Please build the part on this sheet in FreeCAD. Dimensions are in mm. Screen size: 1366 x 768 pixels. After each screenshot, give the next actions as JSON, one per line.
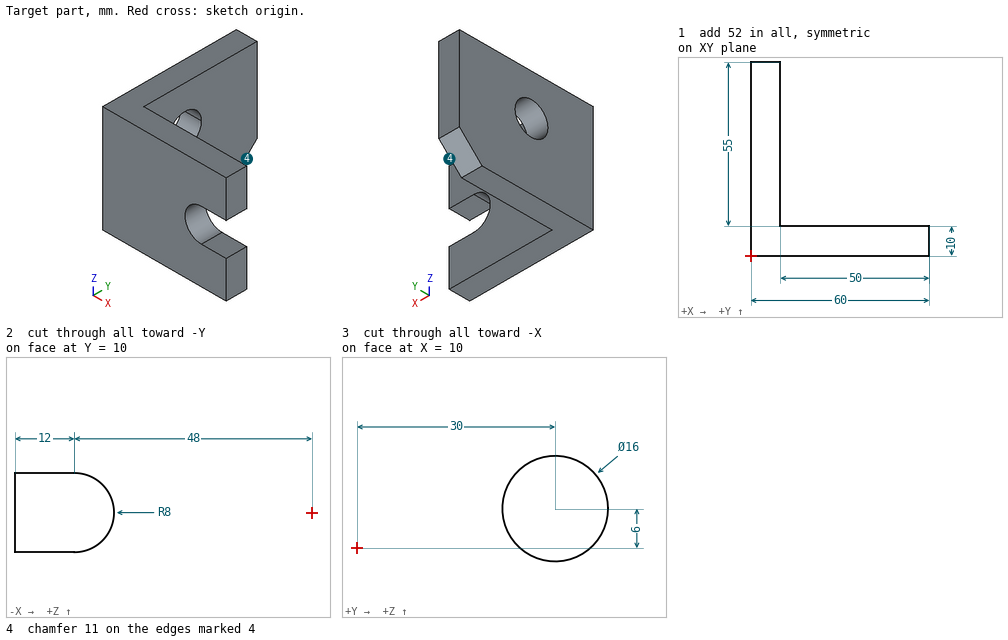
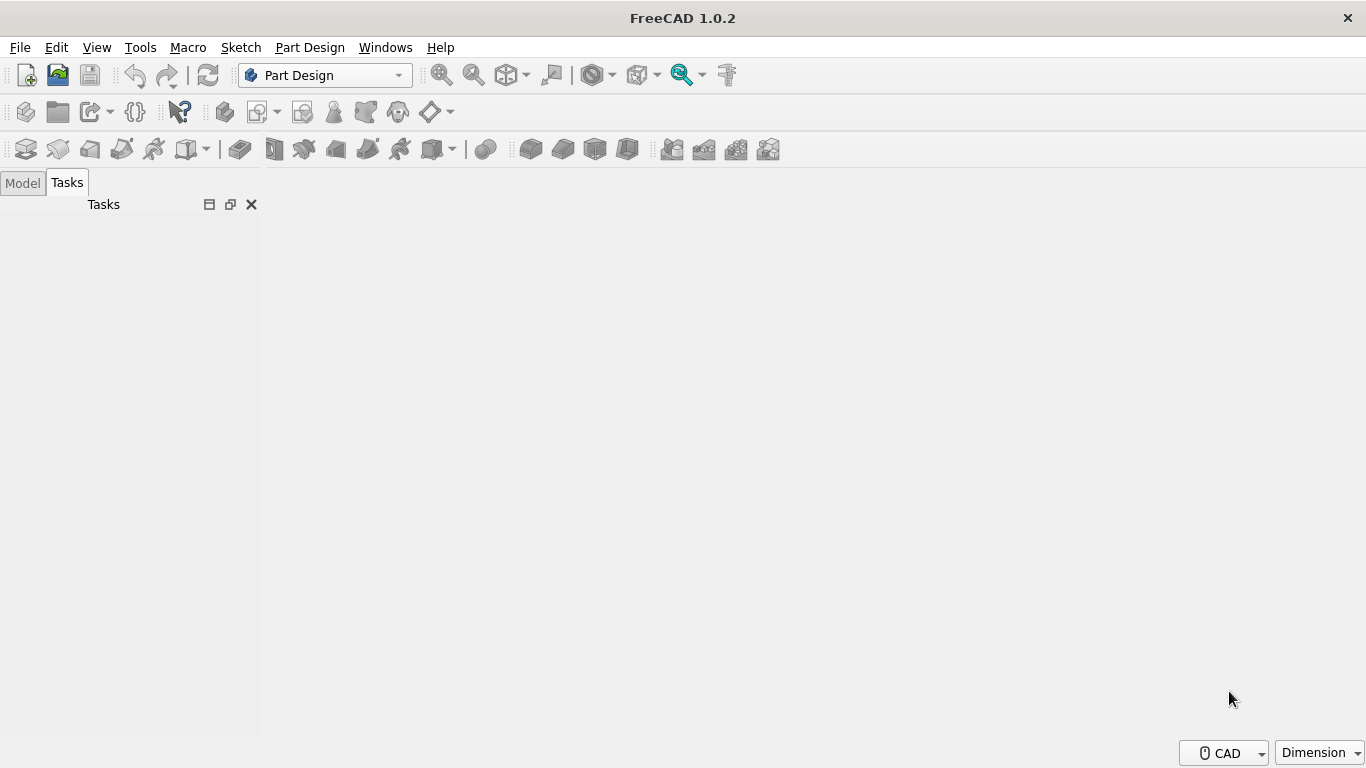
{"action": "left_click", "coordinate": [26, 76]}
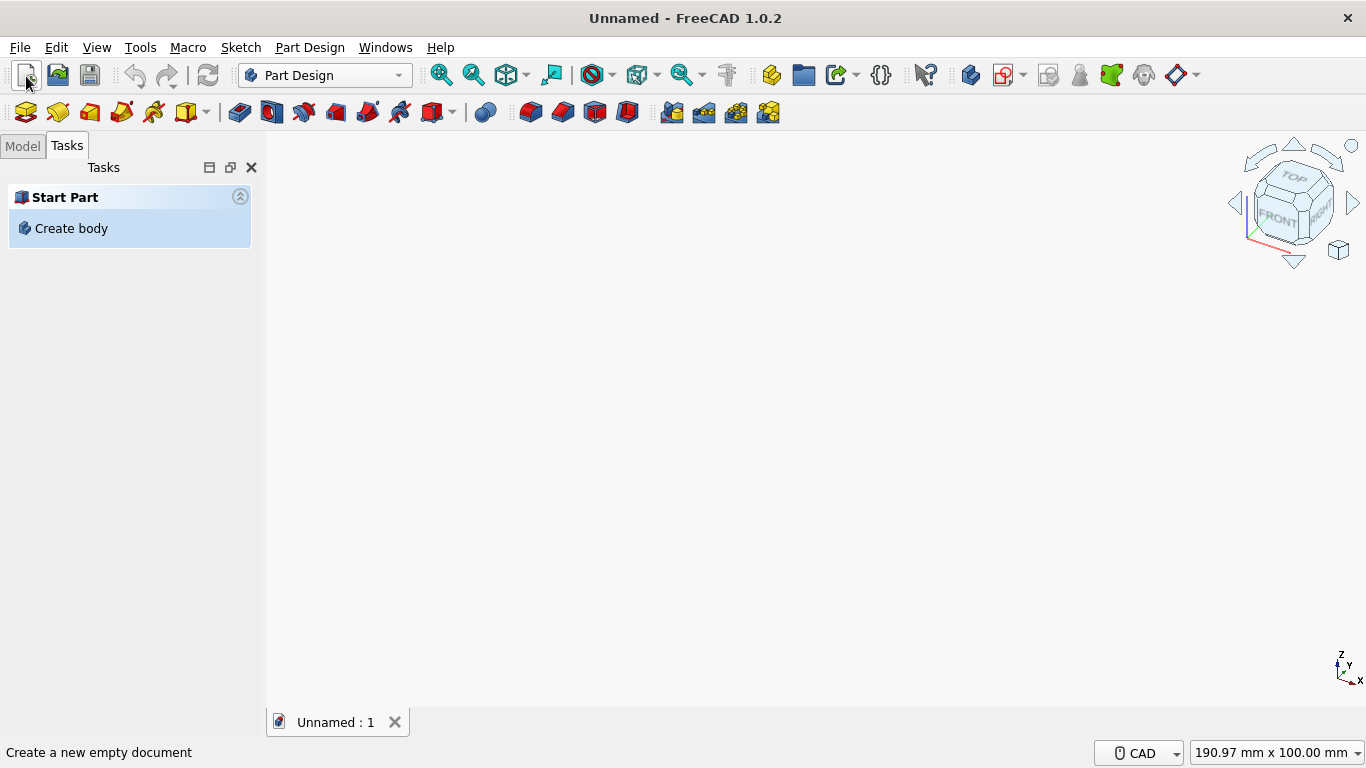
{"action": "left_click", "coordinate": [1004, 76]}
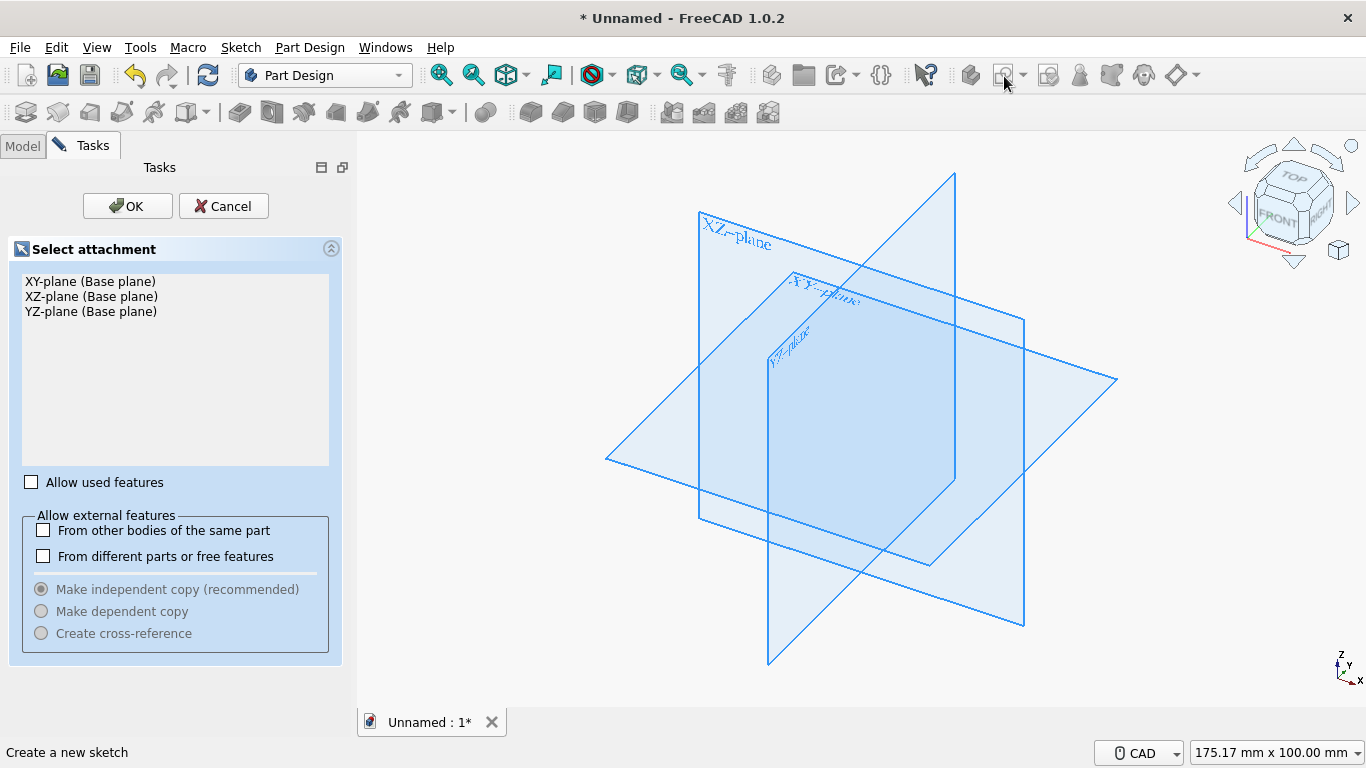
{"action": "left_click", "coordinate": [82, 282]}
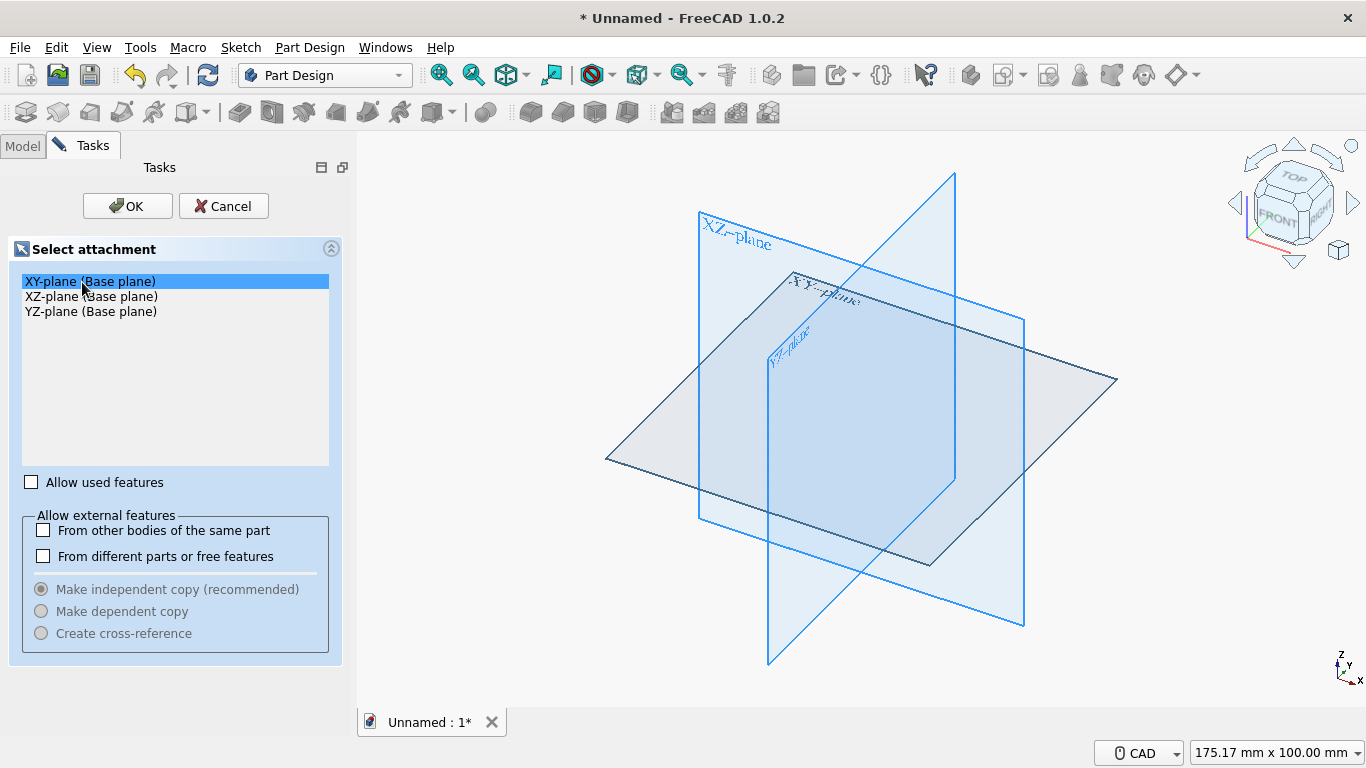
{"action": "left_click", "coordinate": [128, 206]}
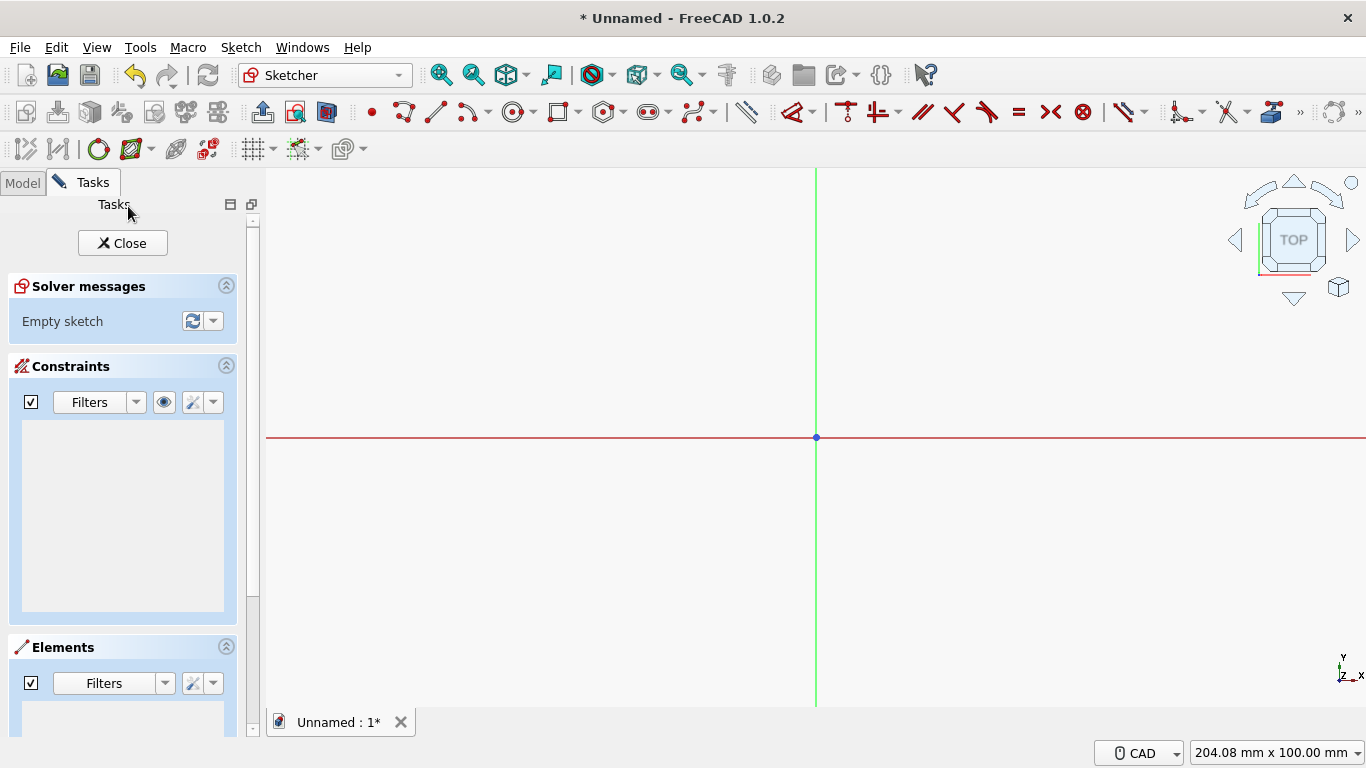
{"action": "scroll", "coordinate": [294, 679], "scroll_direction": "down", "scroll_amount": 2}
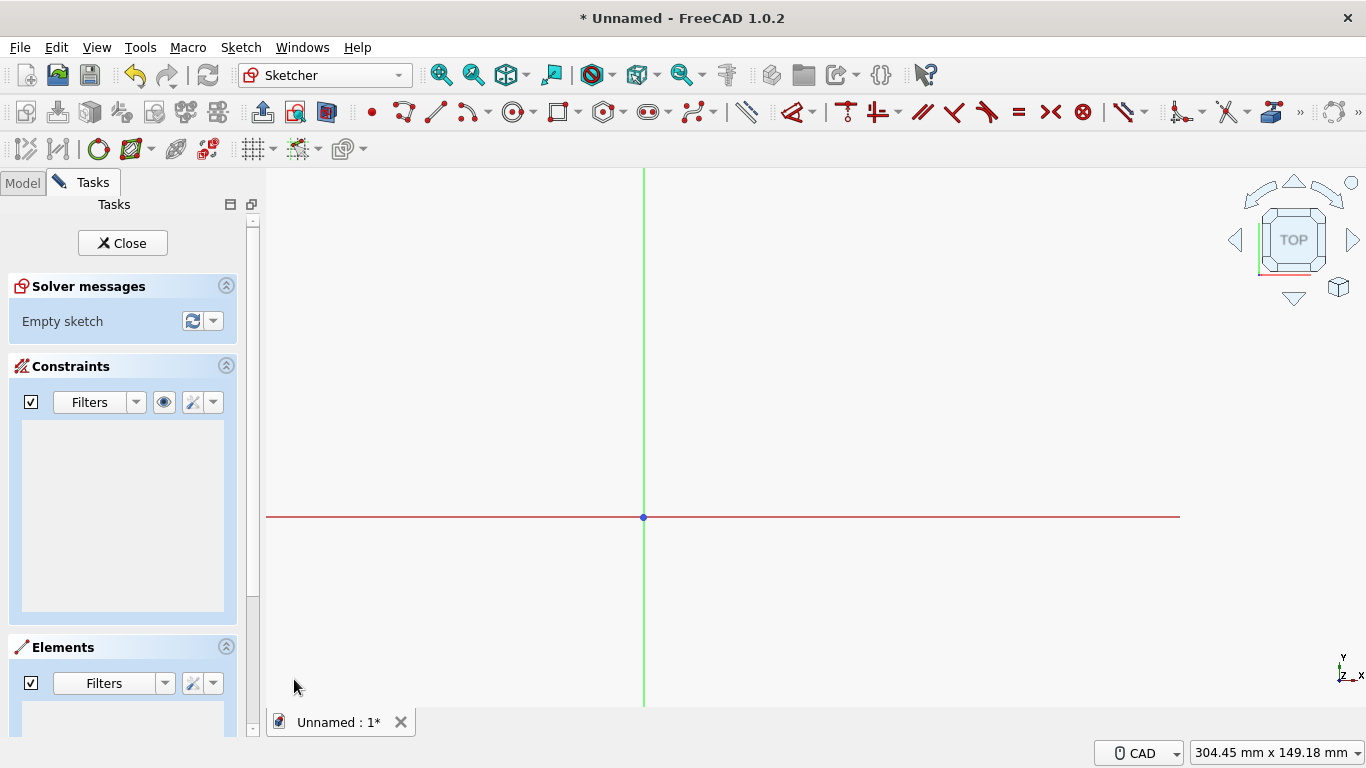
{"action": "scroll", "coordinate": [762, 324], "scroll_direction": "up", "scroll_amount": 2}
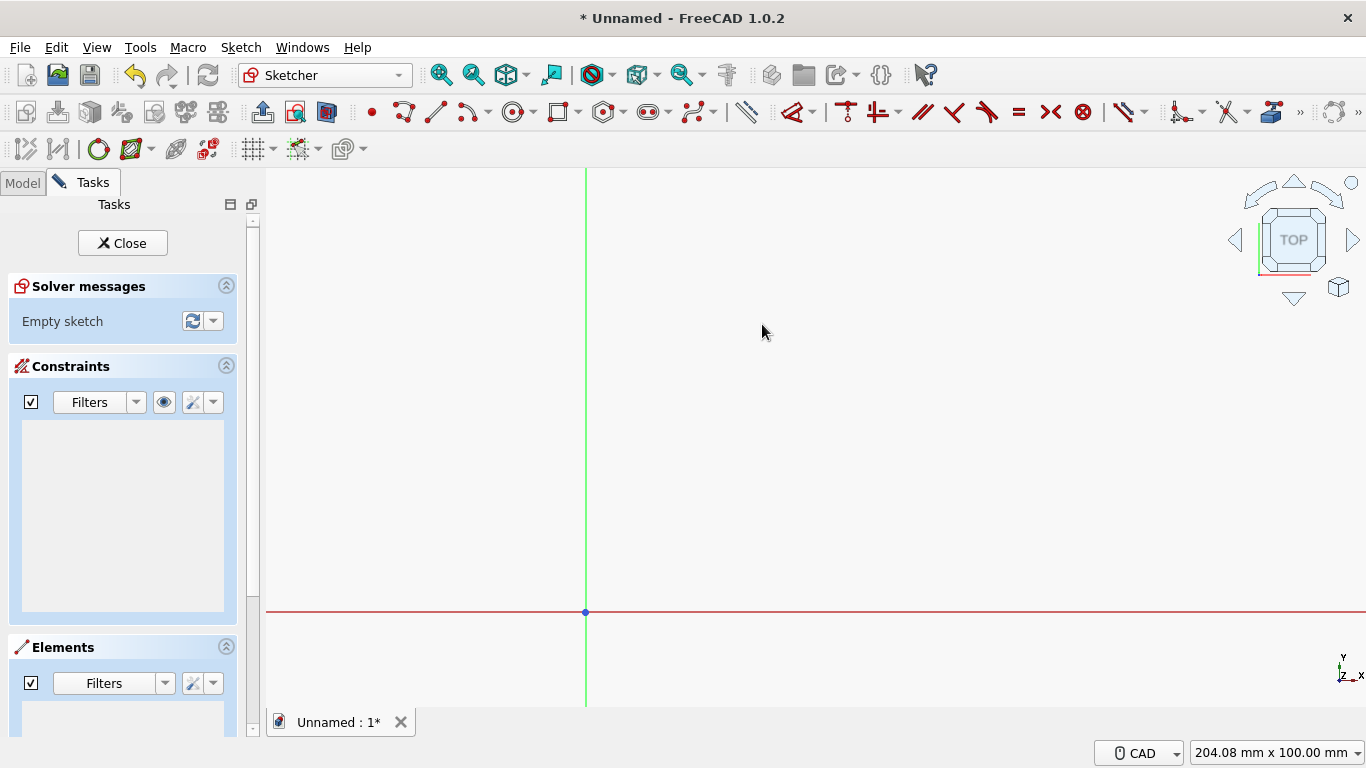
{"action": "left_click", "coordinate": [404, 112]}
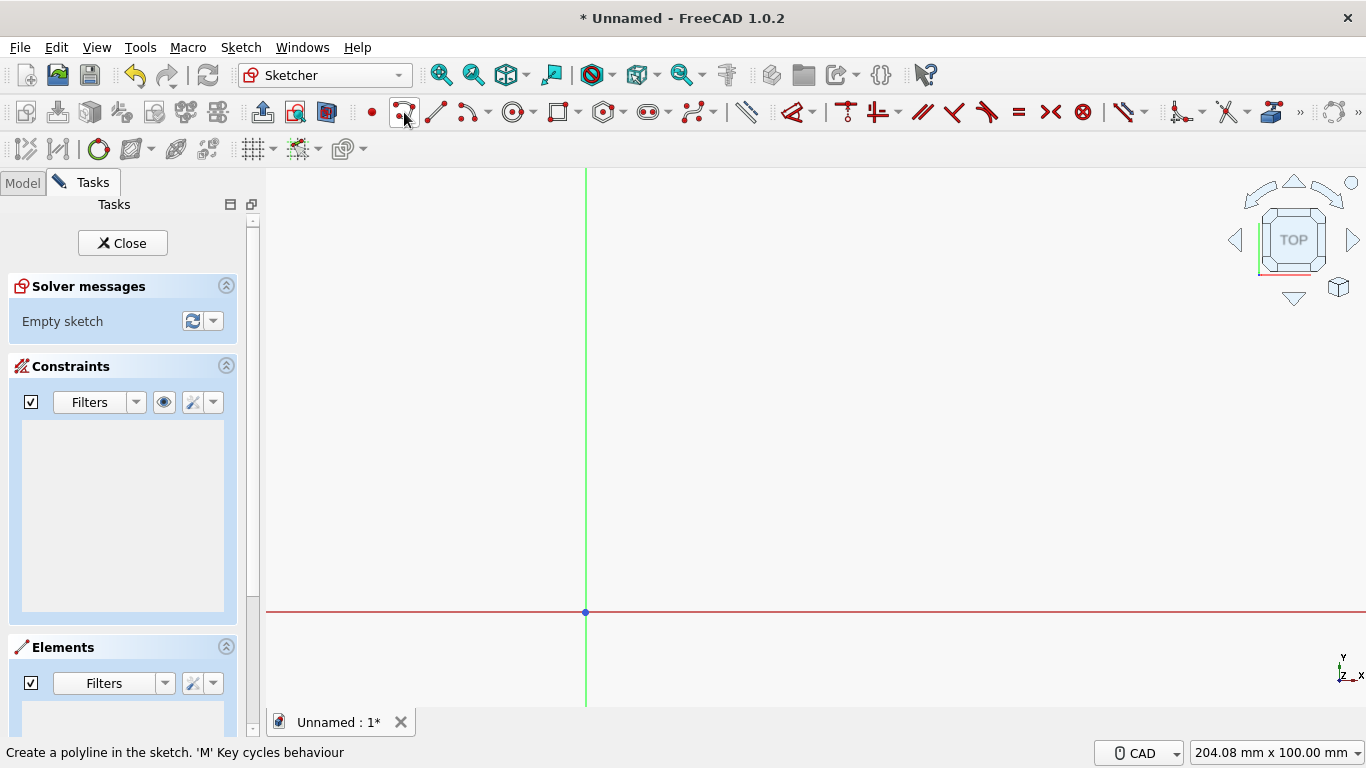
{"action": "left_click", "coordinate": [586, 612]}
{"action": "left_click", "coordinate": [909, 603]}
{"action": "left_click", "coordinate": [909, 559]}
{"action": "left_click", "coordinate": [640, 559]}
{"action": "left_click", "coordinate": [640, 262]}
{"action": "left_click", "coordinate": [595, 262]}
{"action": "left_click", "coordinate": [586, 612]}
{"action": "key", "text": "Escape"}
{"action": "key", "text": "Escape"}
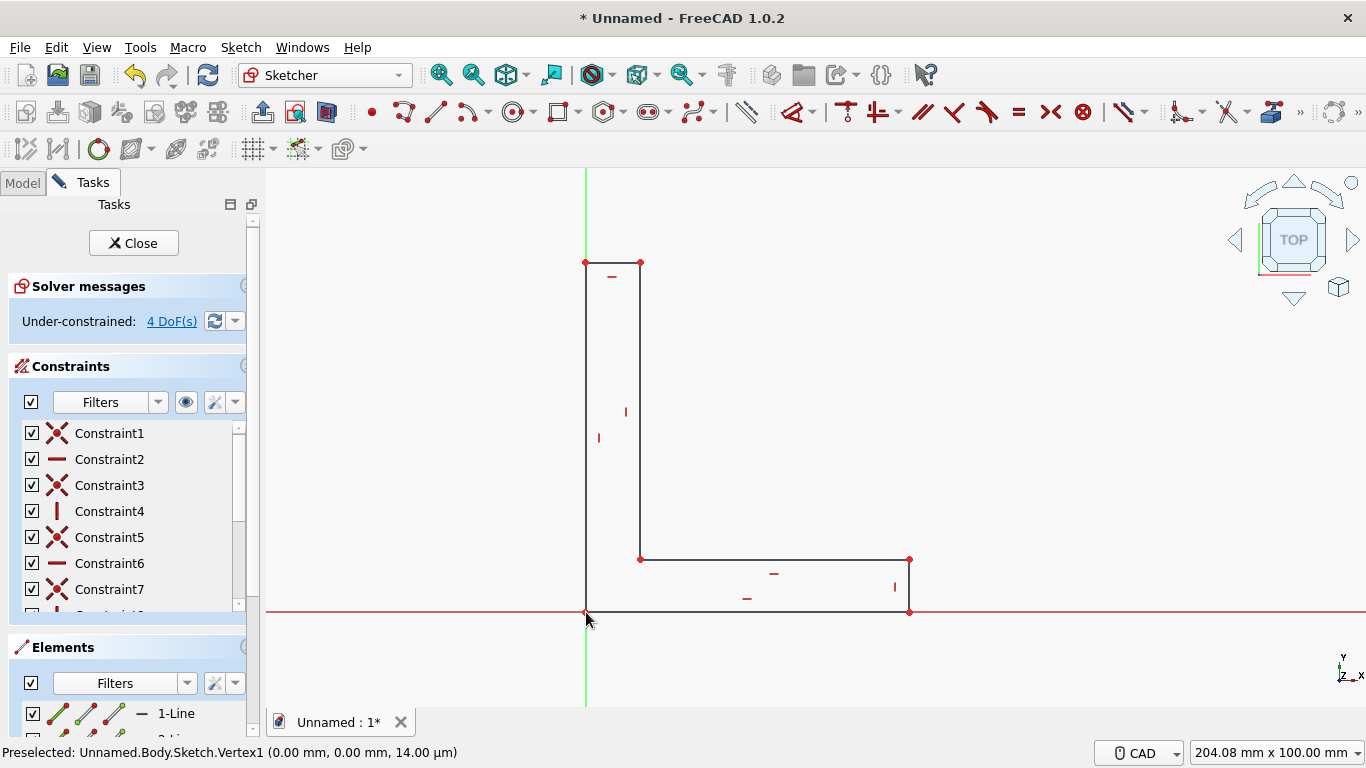
{"action": "left_click", "coordinate": [792, 112]}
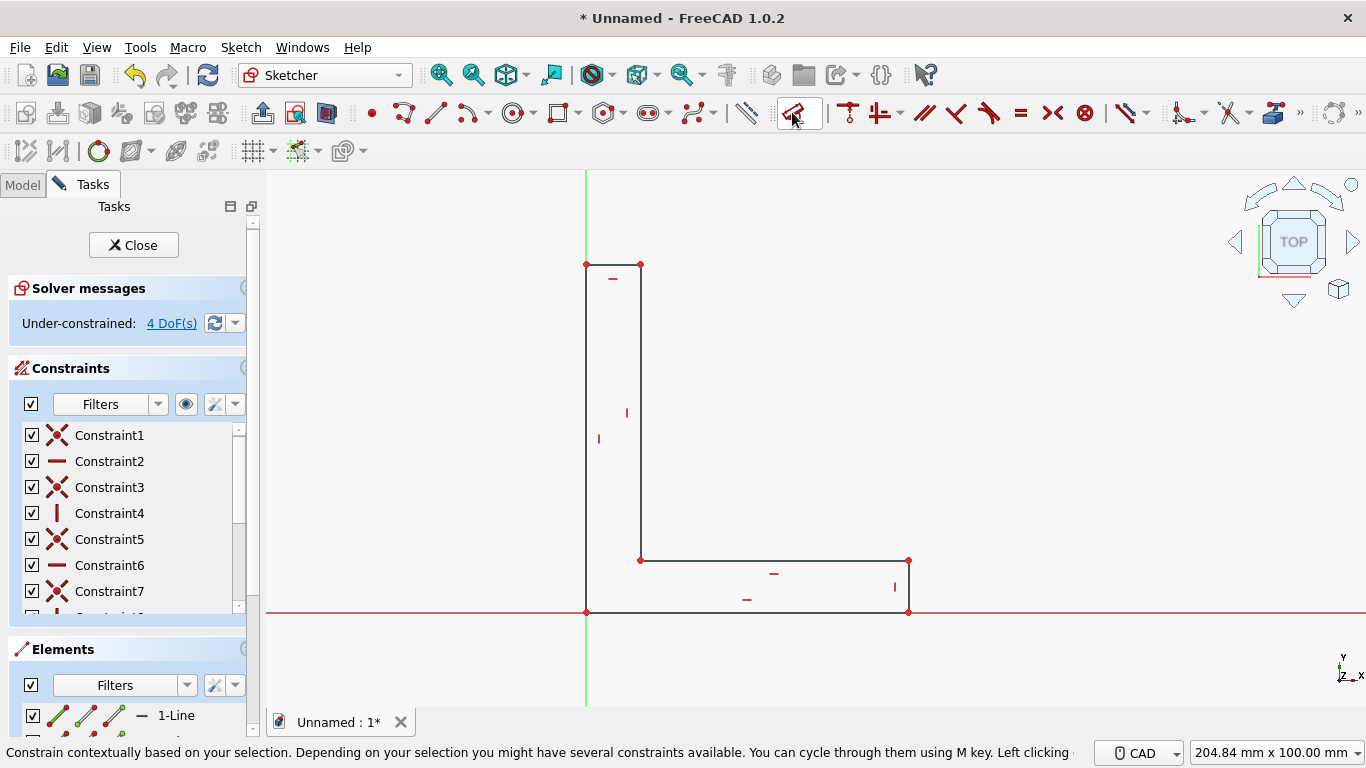
{"action": "left_click", "coordinate": [683, 613]}
{"action": "left_click", "coordinate": [748, 647]}